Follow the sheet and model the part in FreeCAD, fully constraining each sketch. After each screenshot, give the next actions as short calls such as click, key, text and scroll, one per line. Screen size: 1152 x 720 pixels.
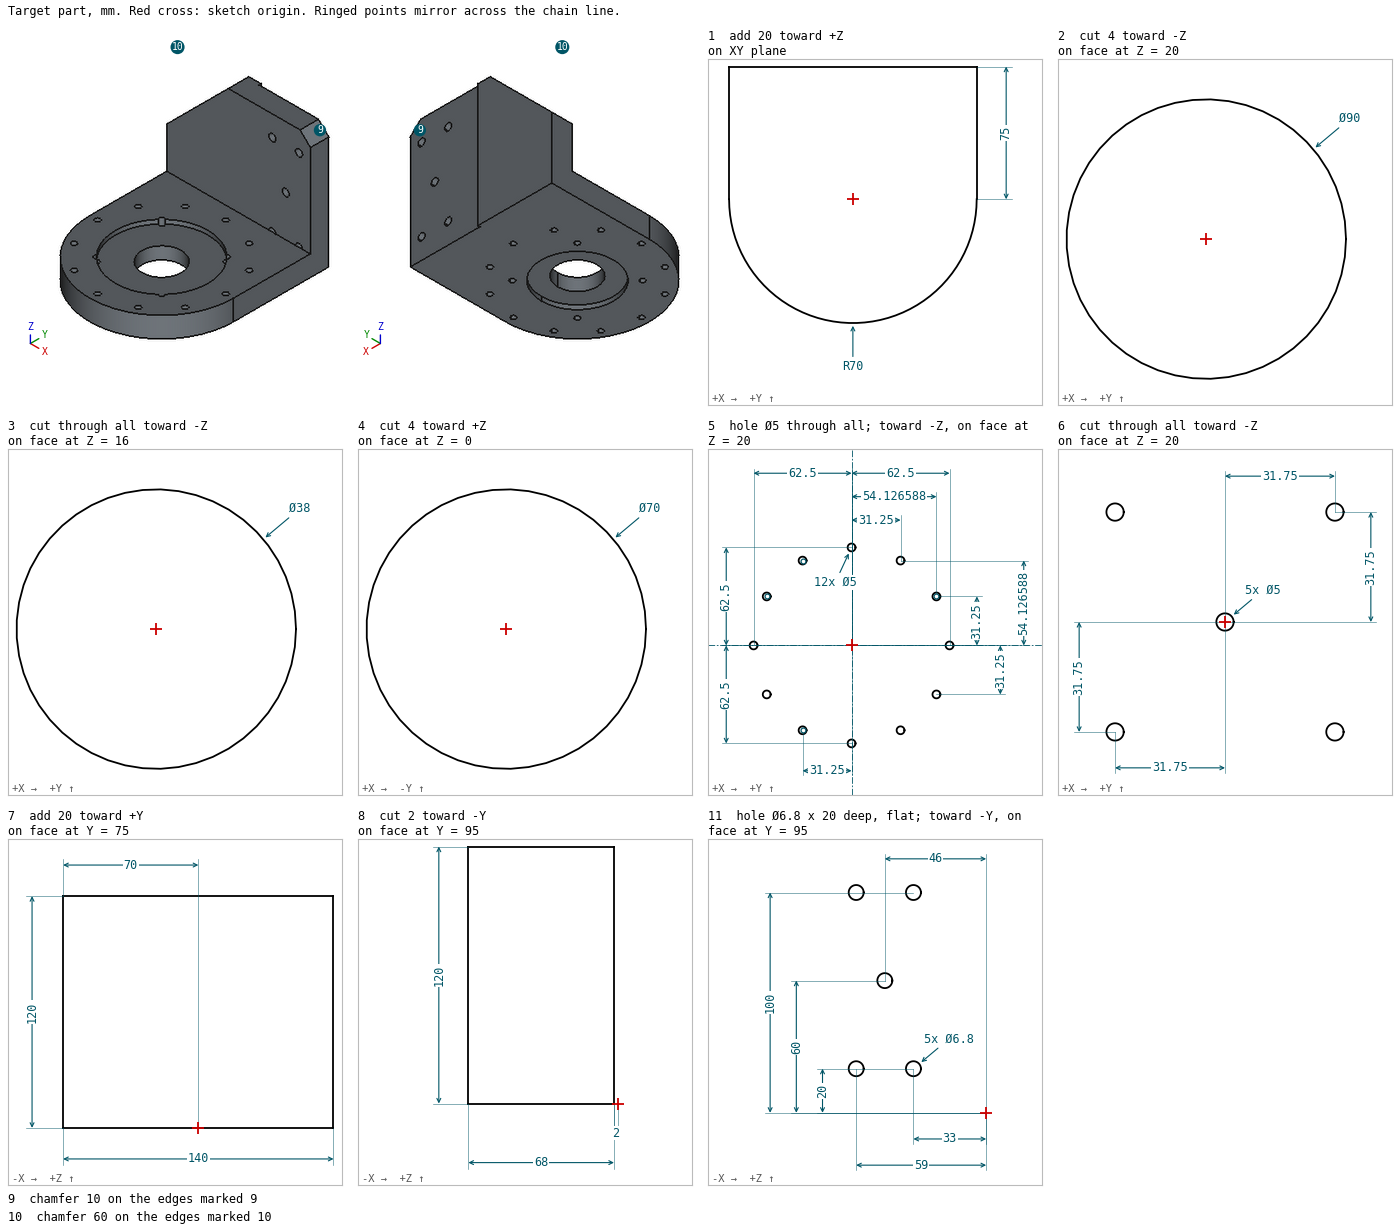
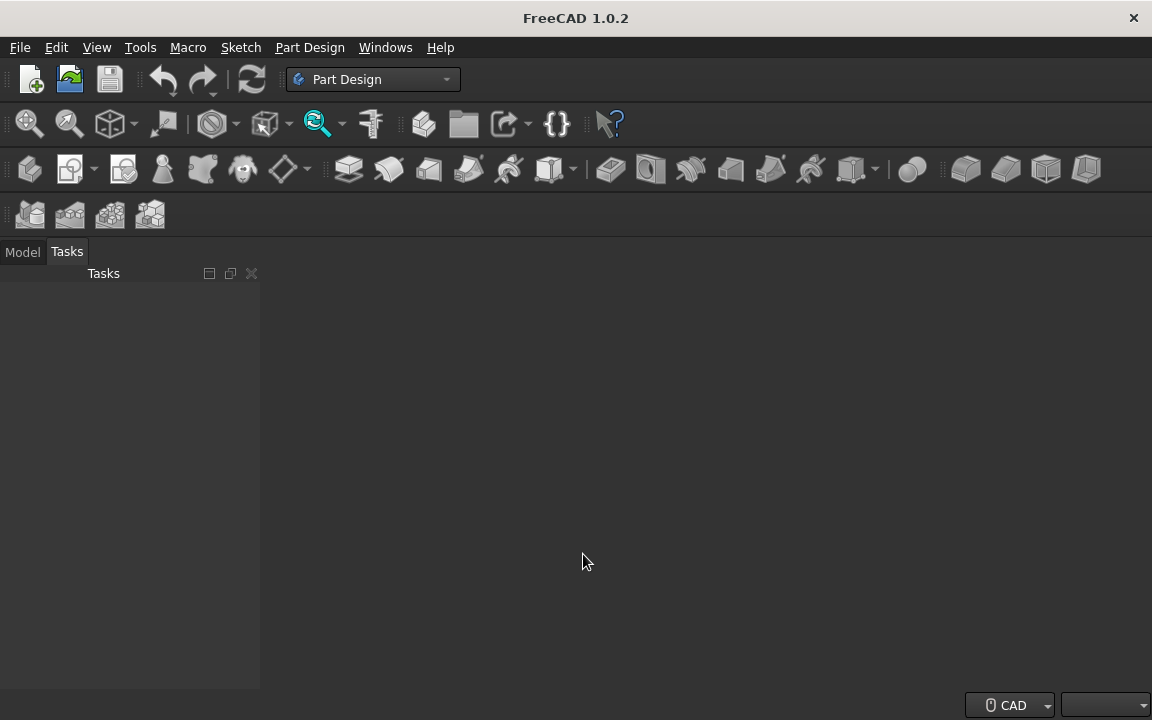
click(30, 80)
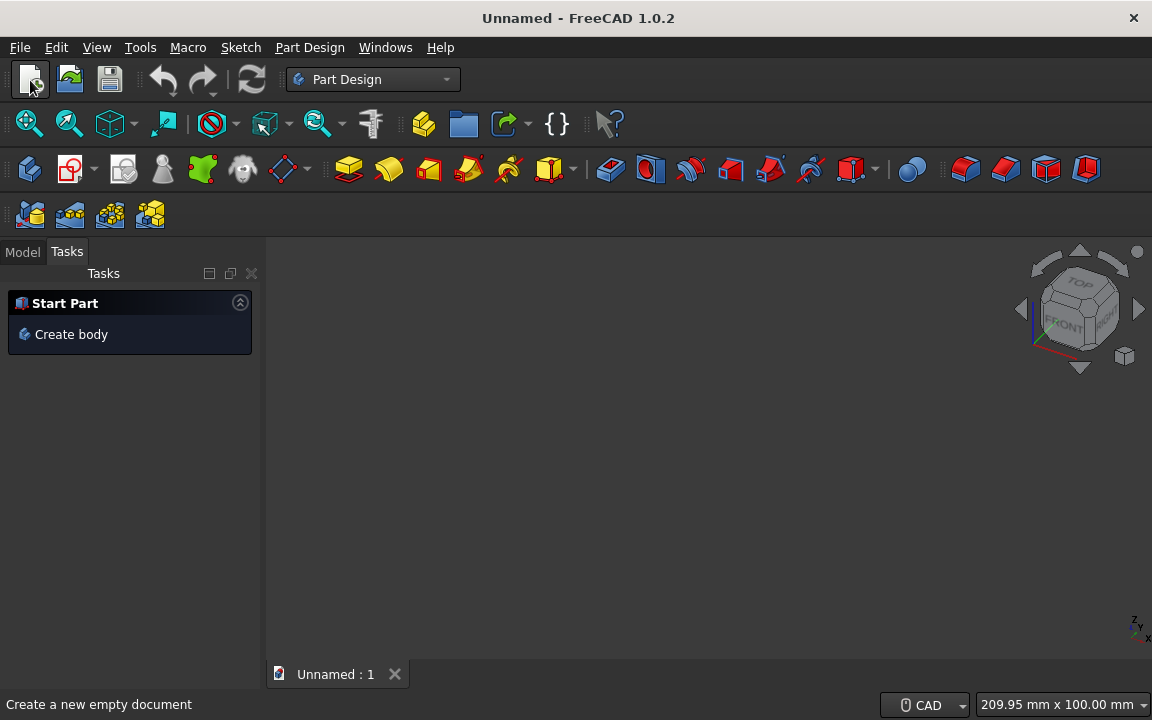
click(70, 170)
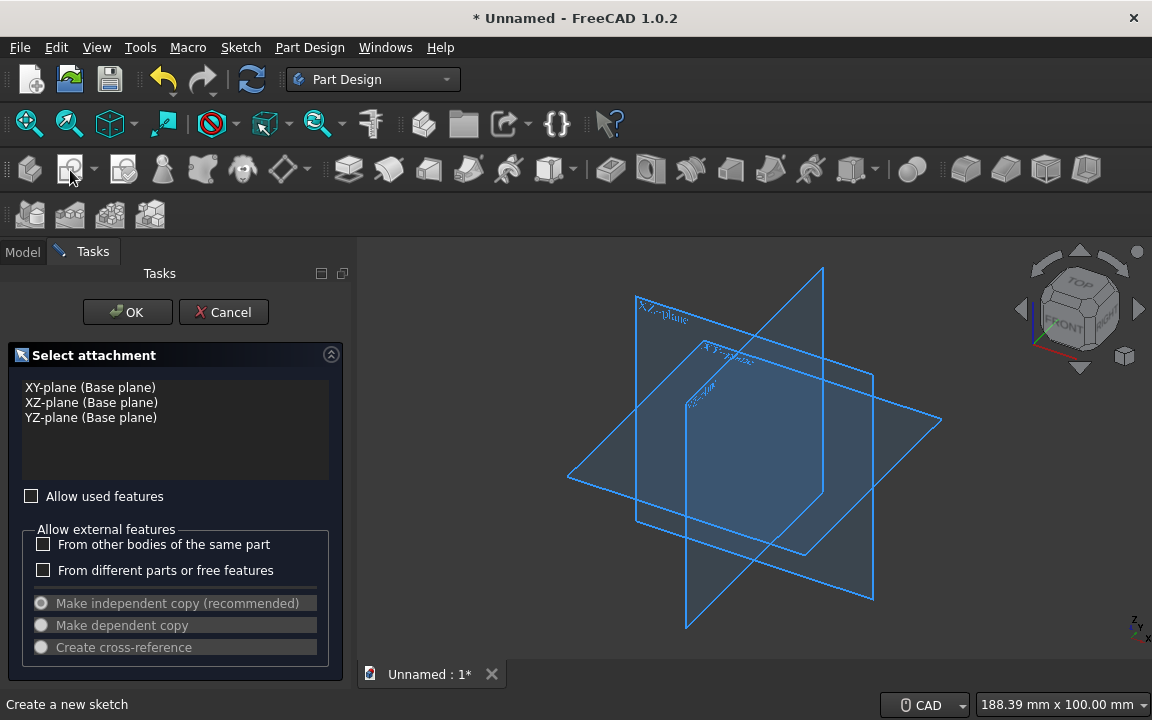
click(82, 388)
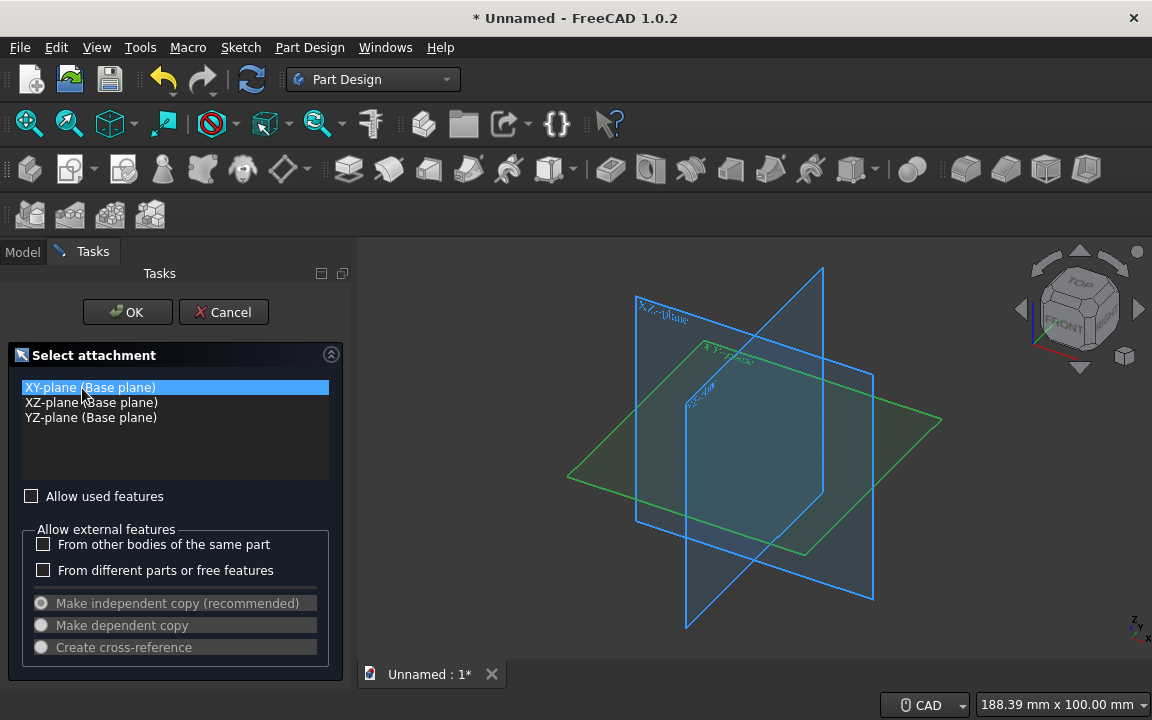
click(128, 312)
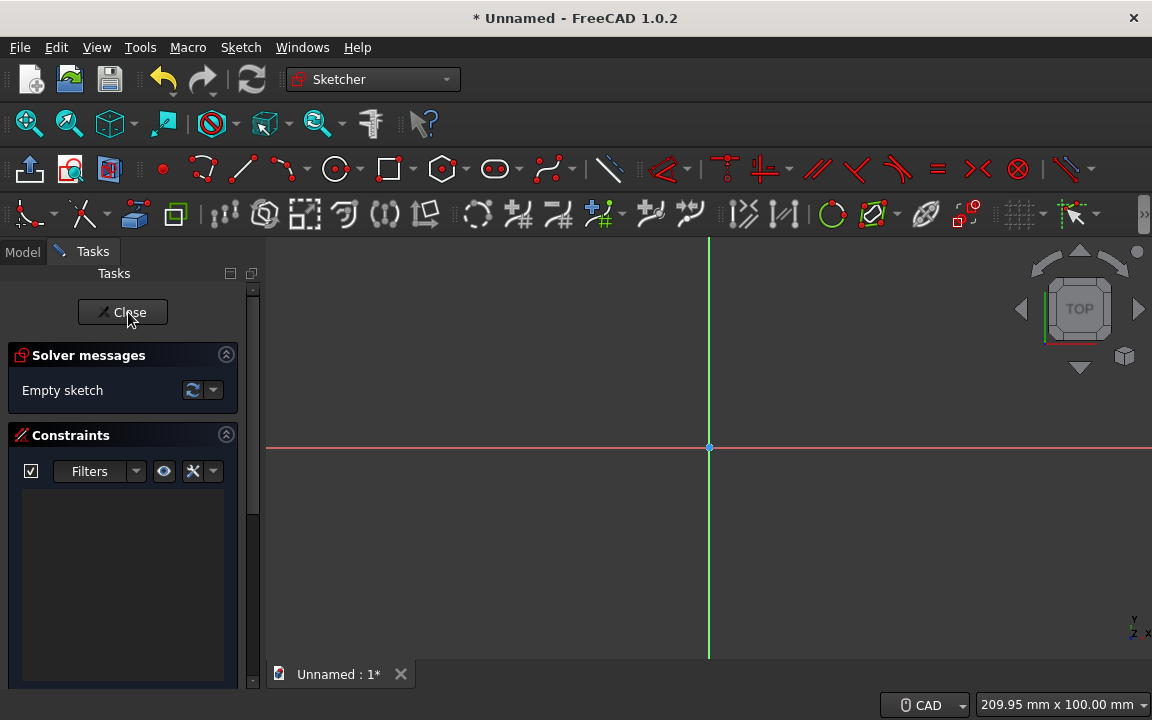
scroll(585, 457, down, 4)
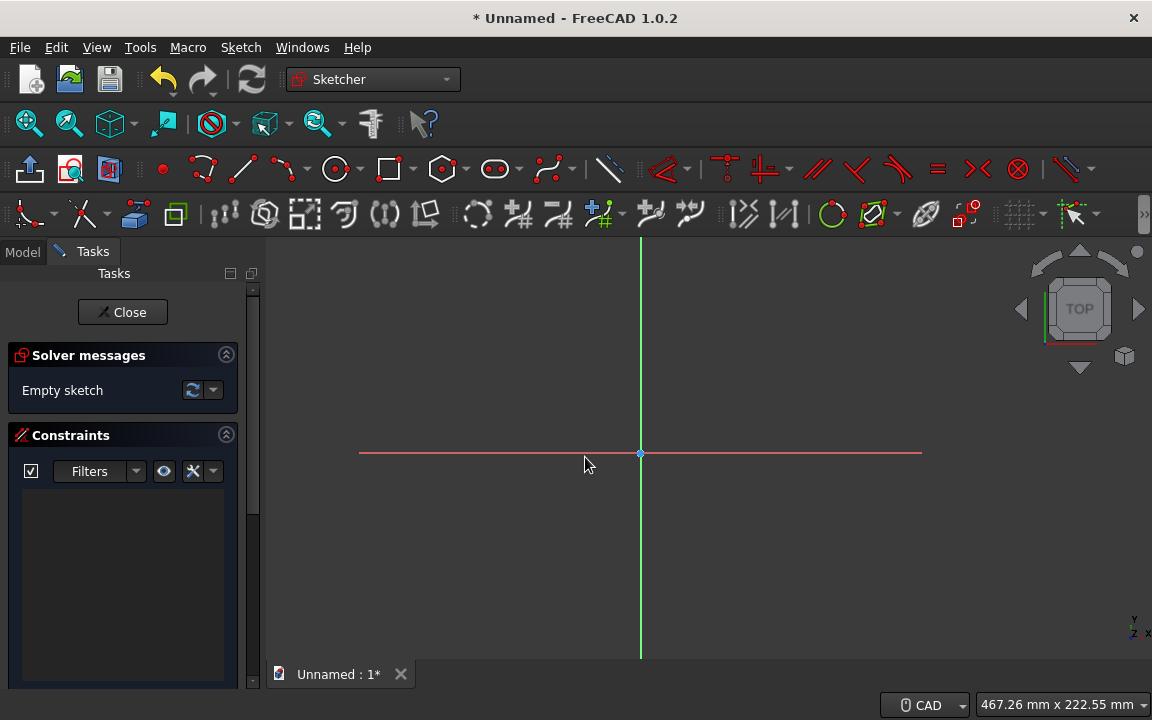
key(g)
key(m)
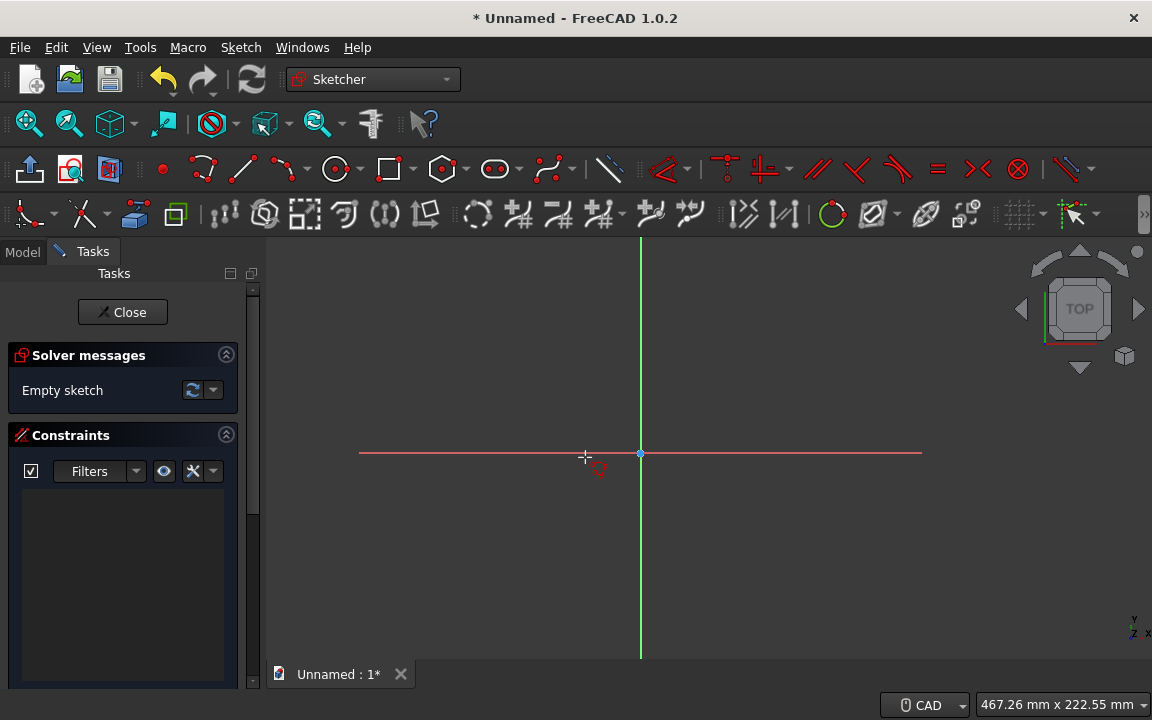
click(774, 453)
click(774, 311)
click(508, 311)
click(508, 453)
right_click(508, 453)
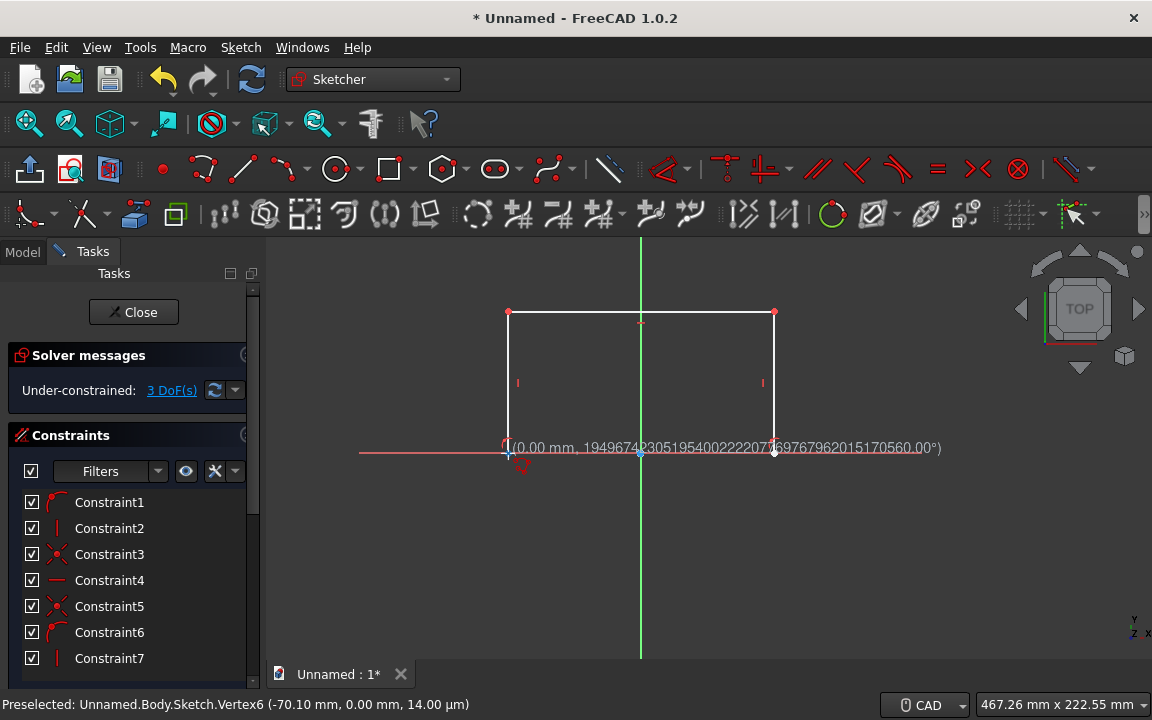
key(g)
key(3)
key(a)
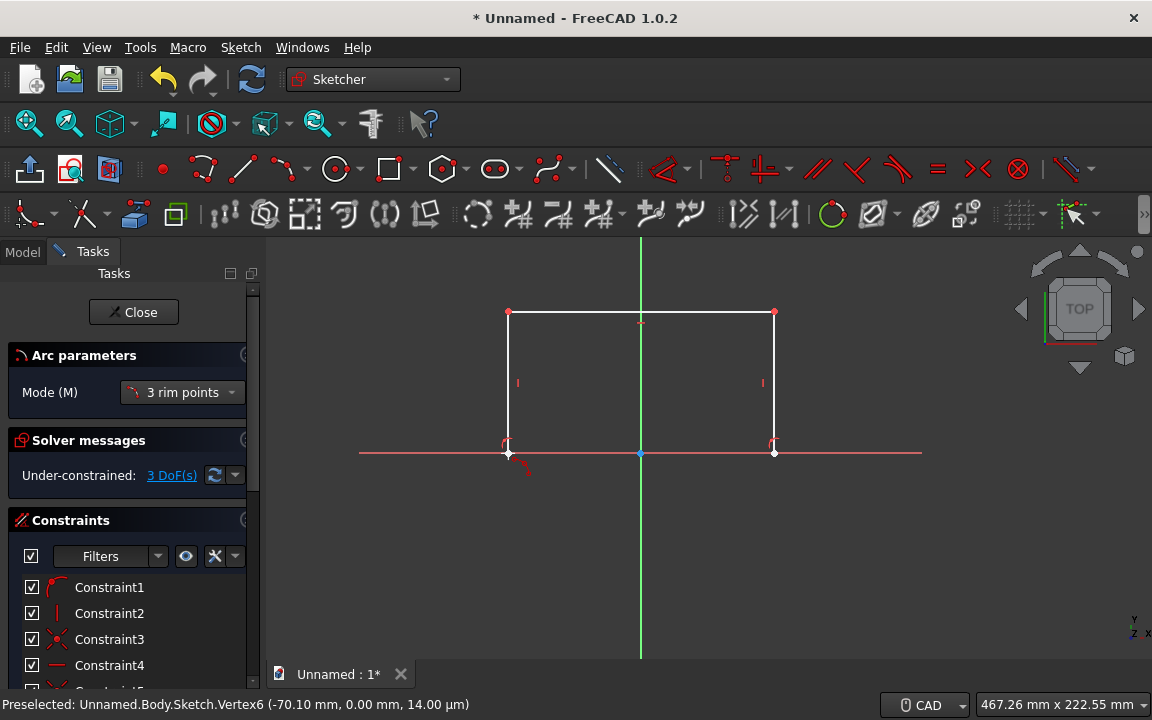
click(508, 453)
click(774, 453)
click(600, 579)
key(Escape)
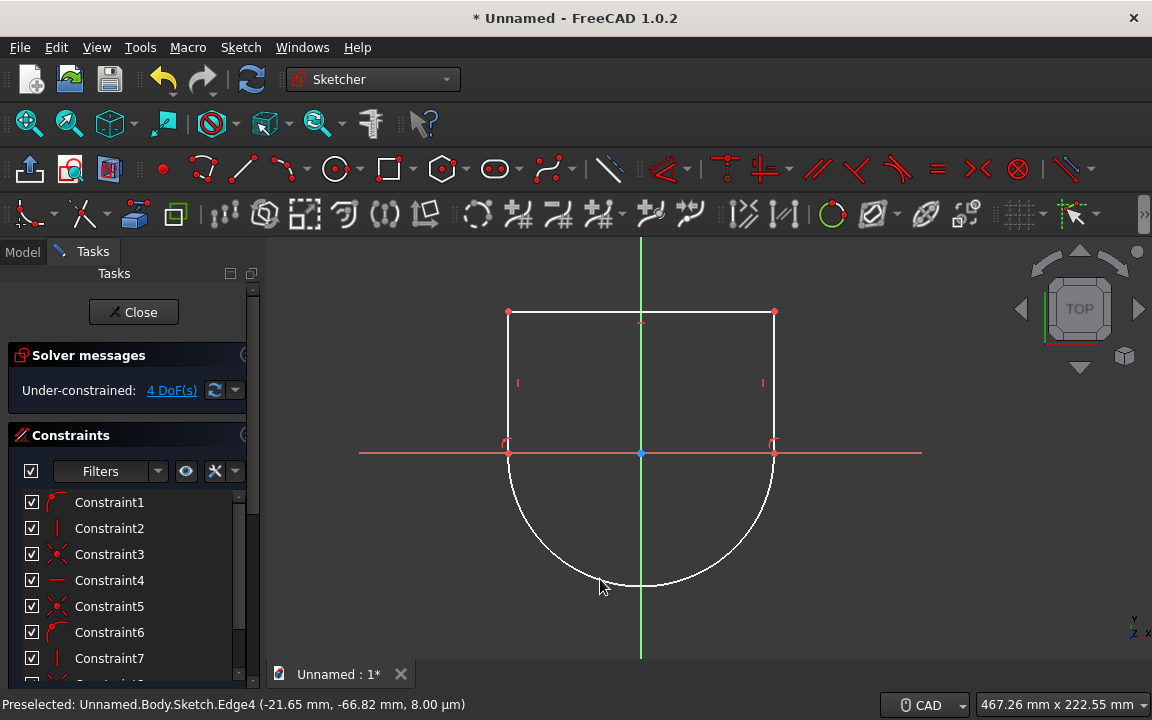
drag(631, 443, 651, 463)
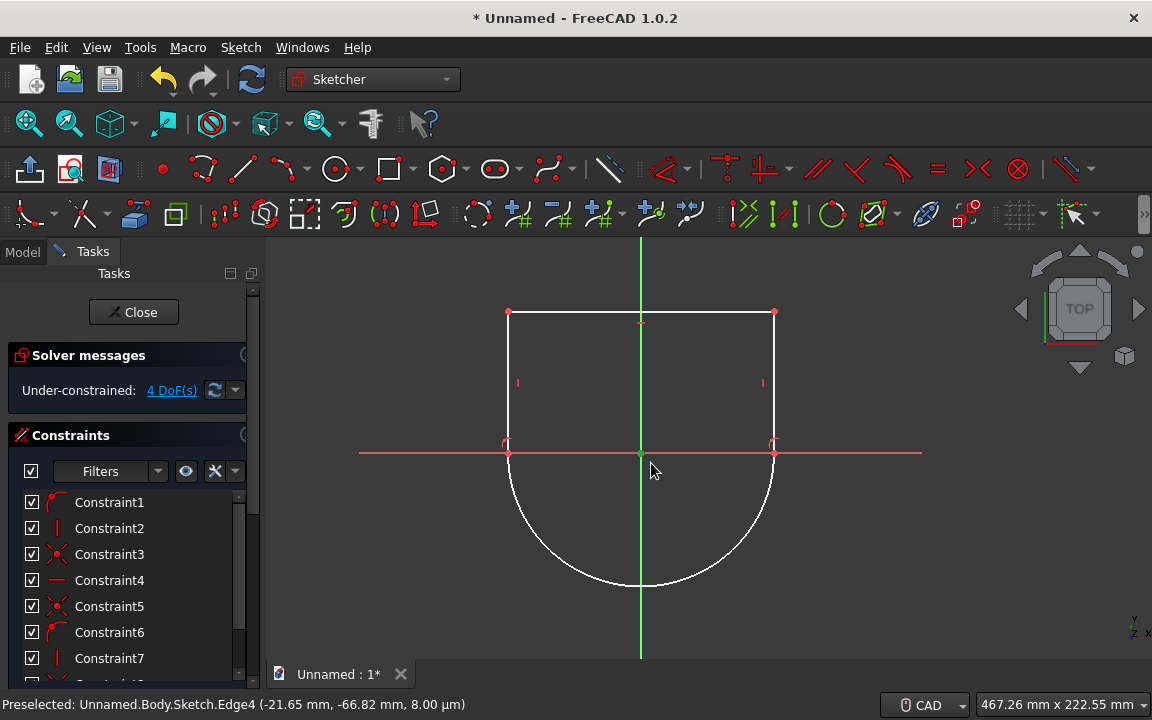
click(726, 170)